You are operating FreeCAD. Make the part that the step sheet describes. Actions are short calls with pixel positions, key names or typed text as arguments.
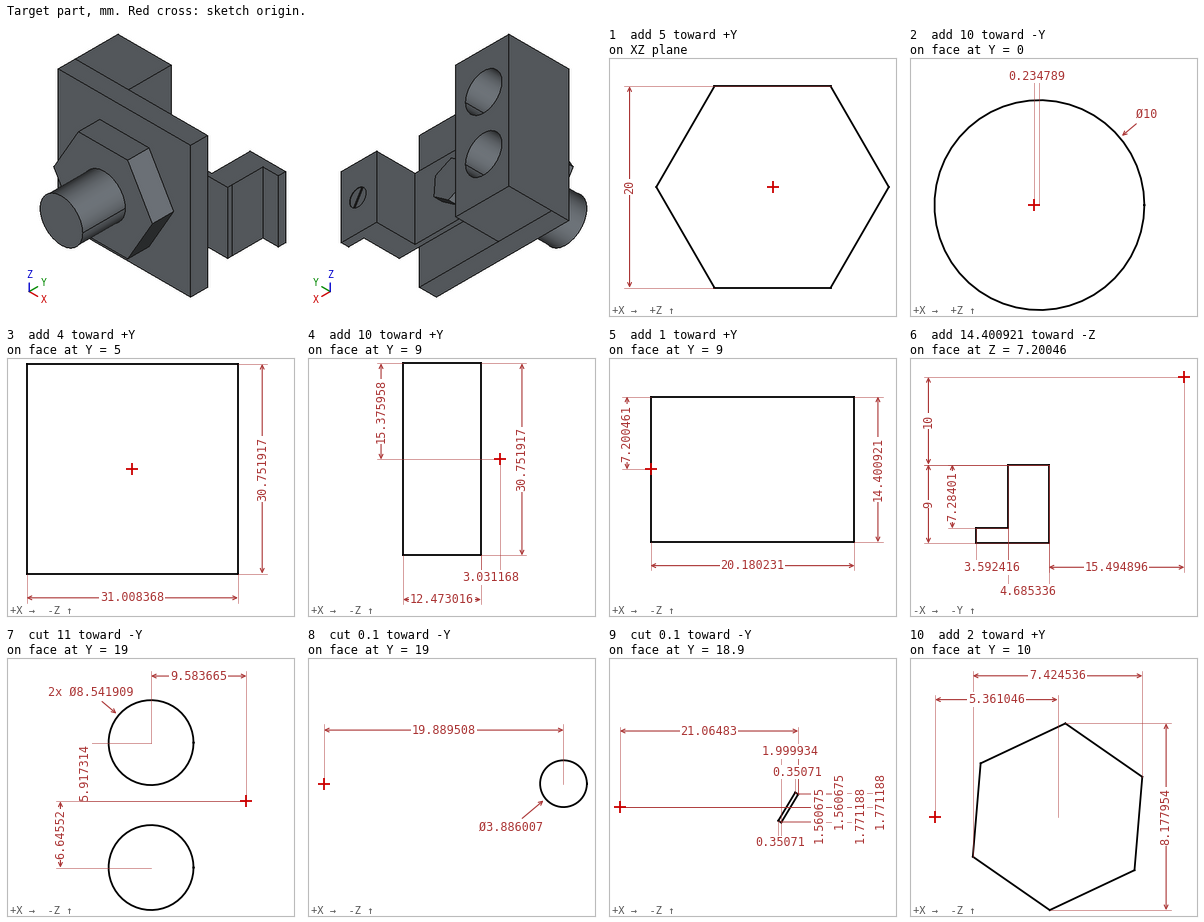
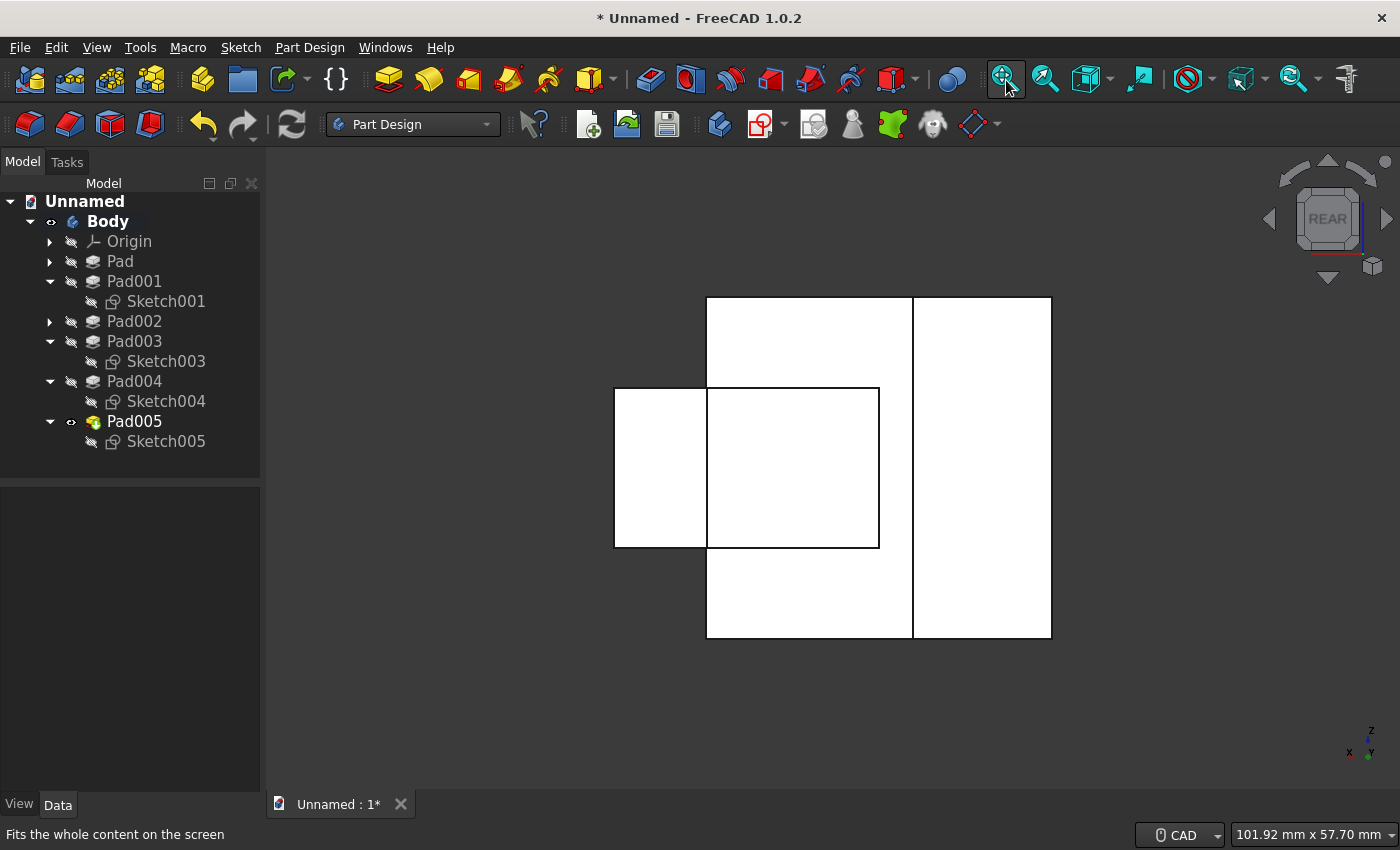
click(982, 516)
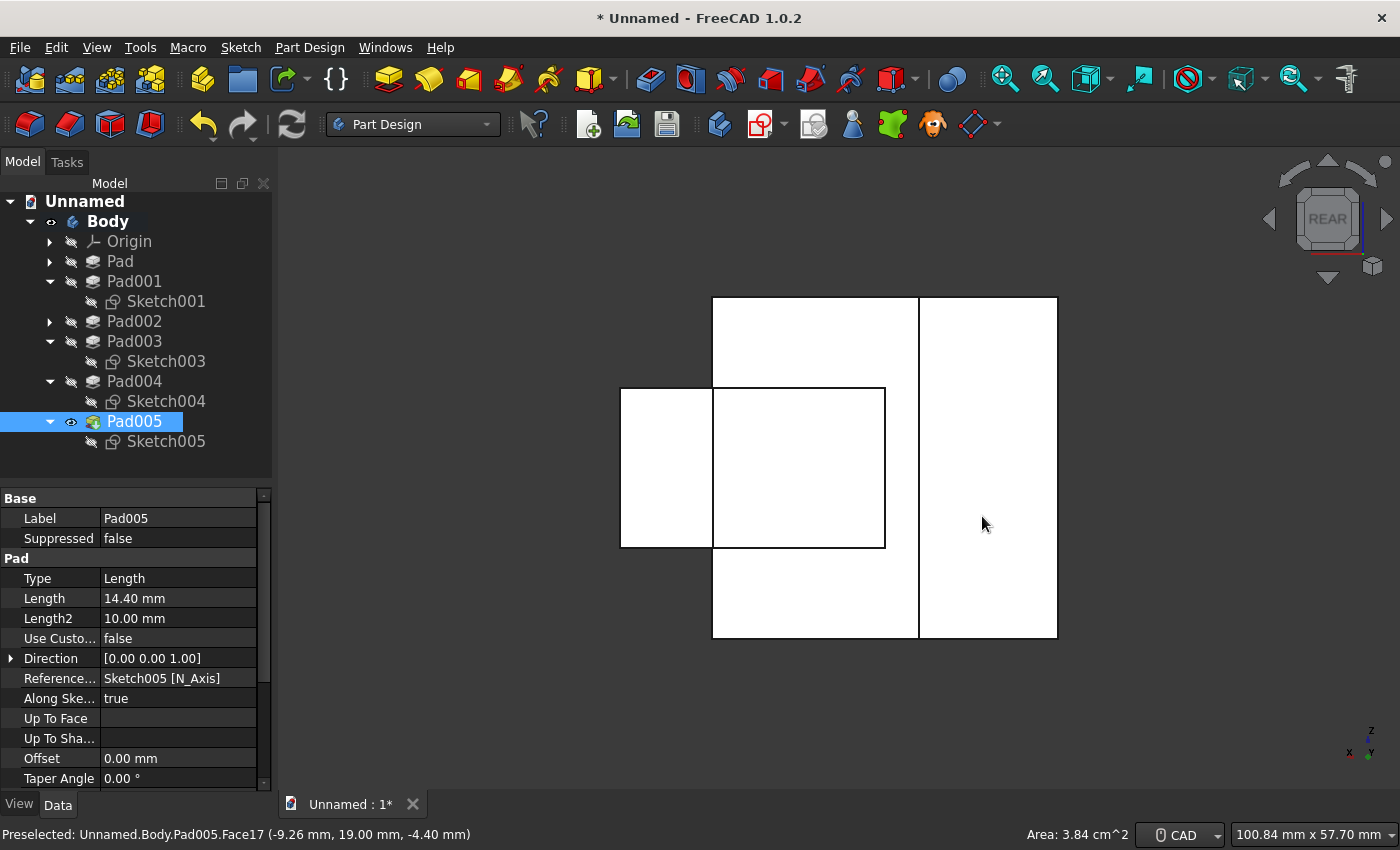
click(760, 124)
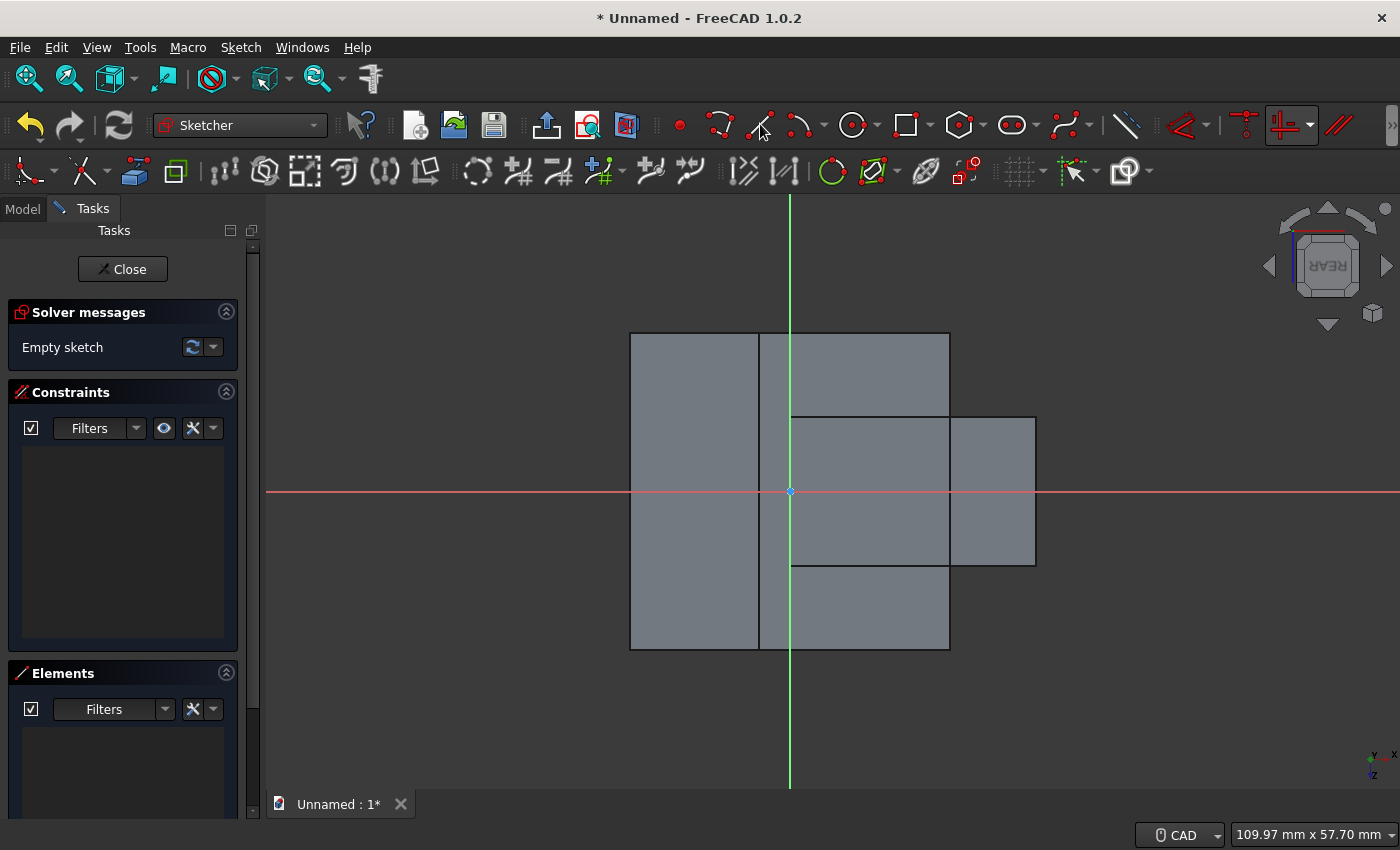
scroll(664, 500, up, 3)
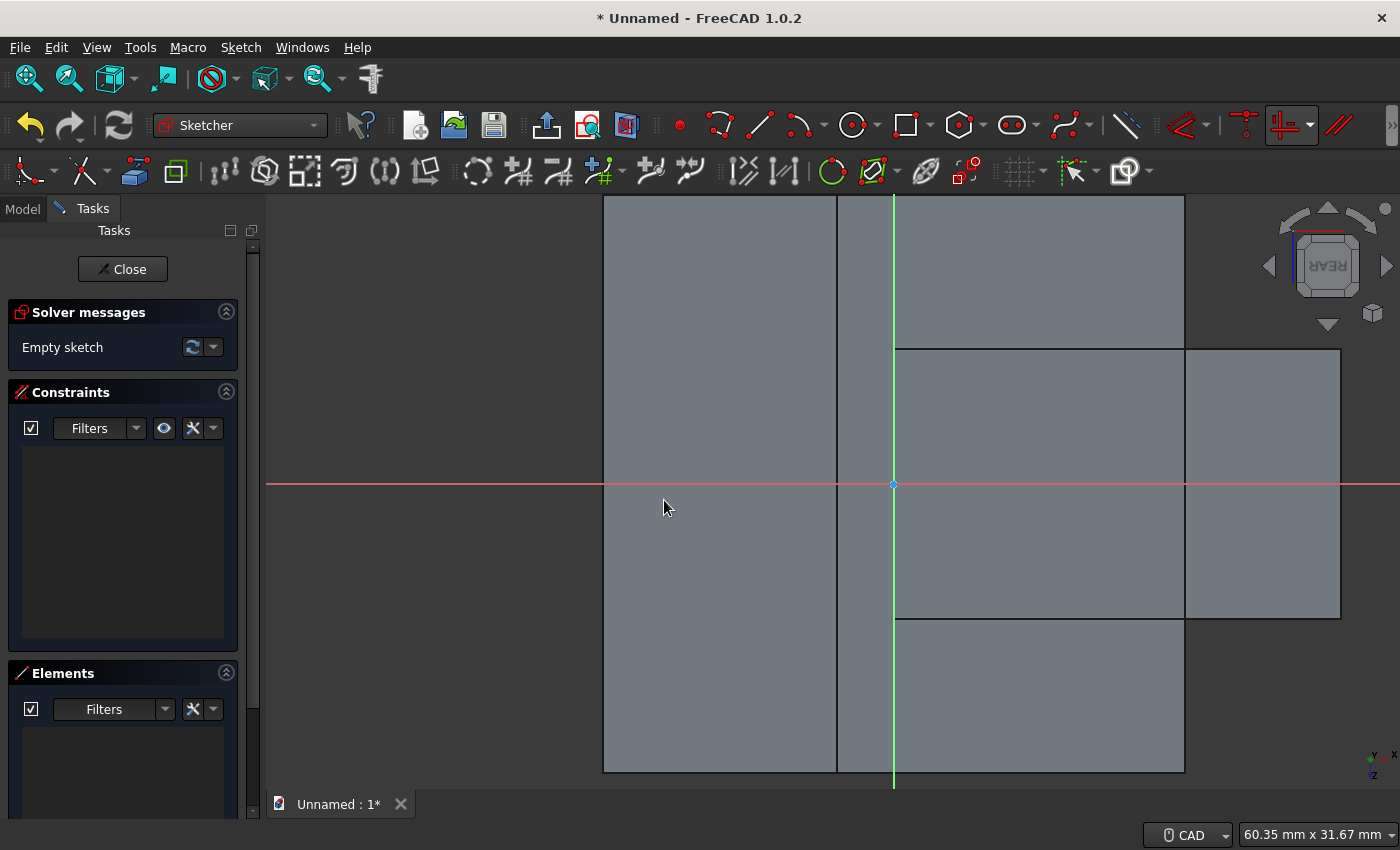
click(854, 126)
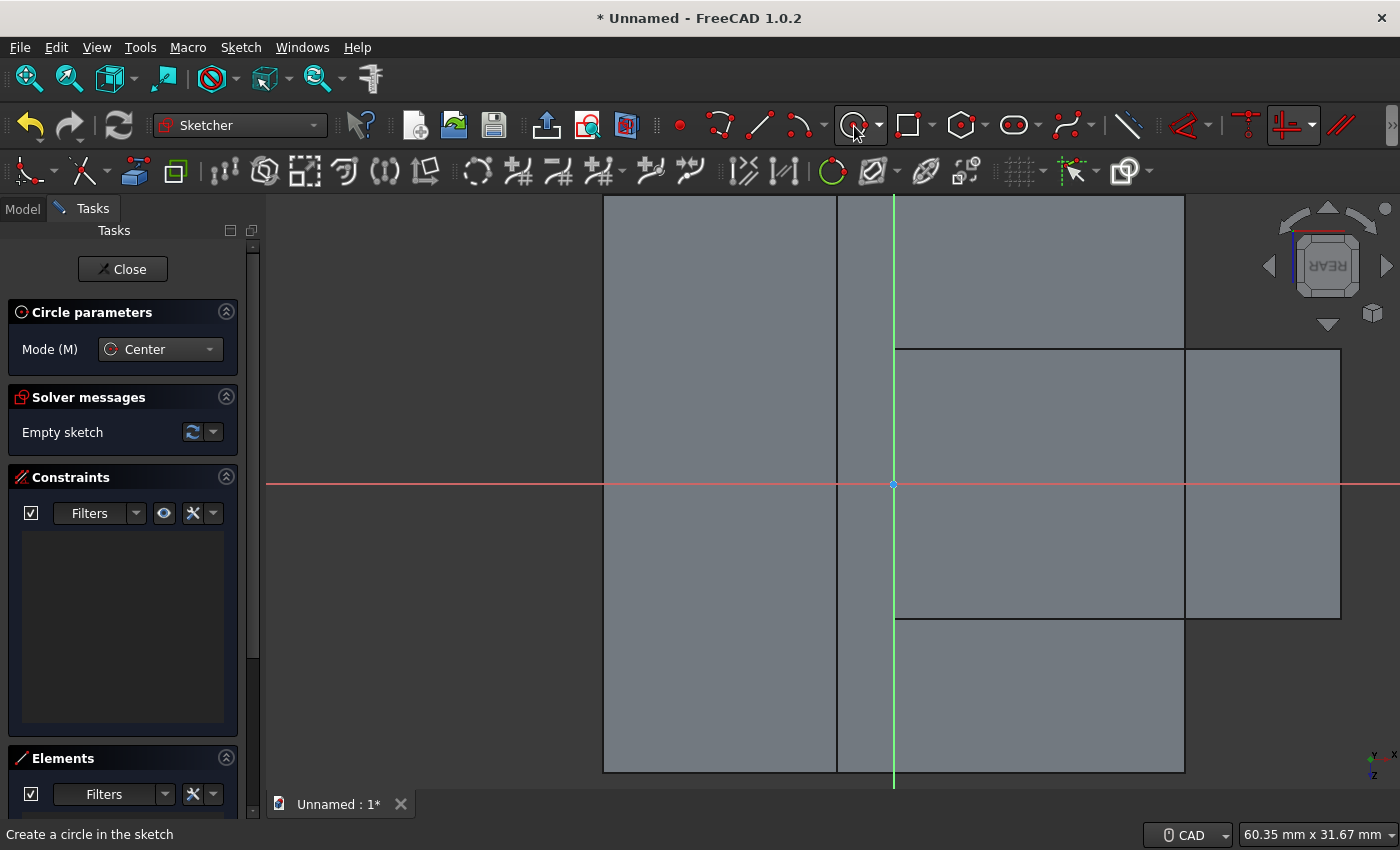
click(714, 373)
move(771, 316)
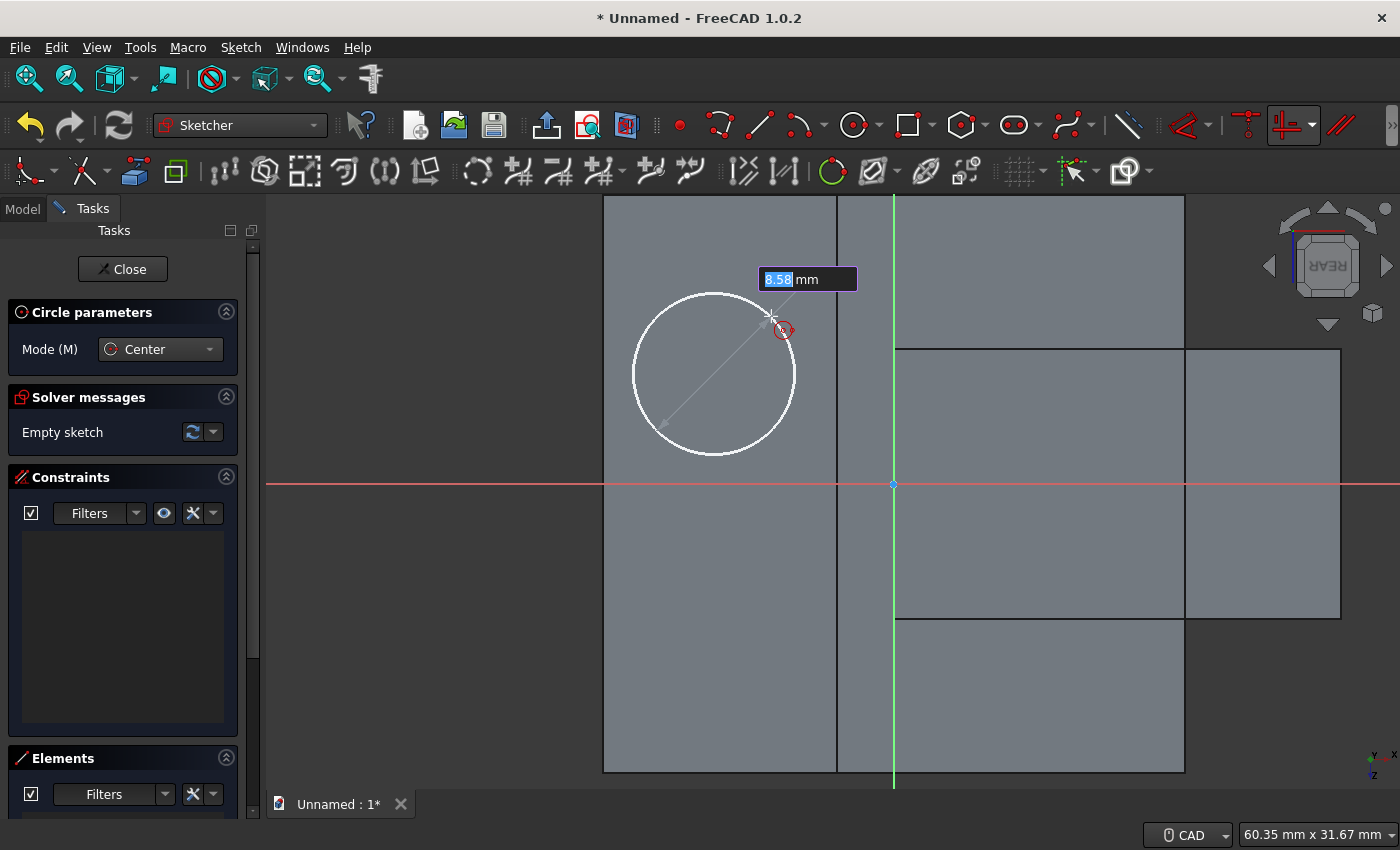
text(8.541909)
key(Return)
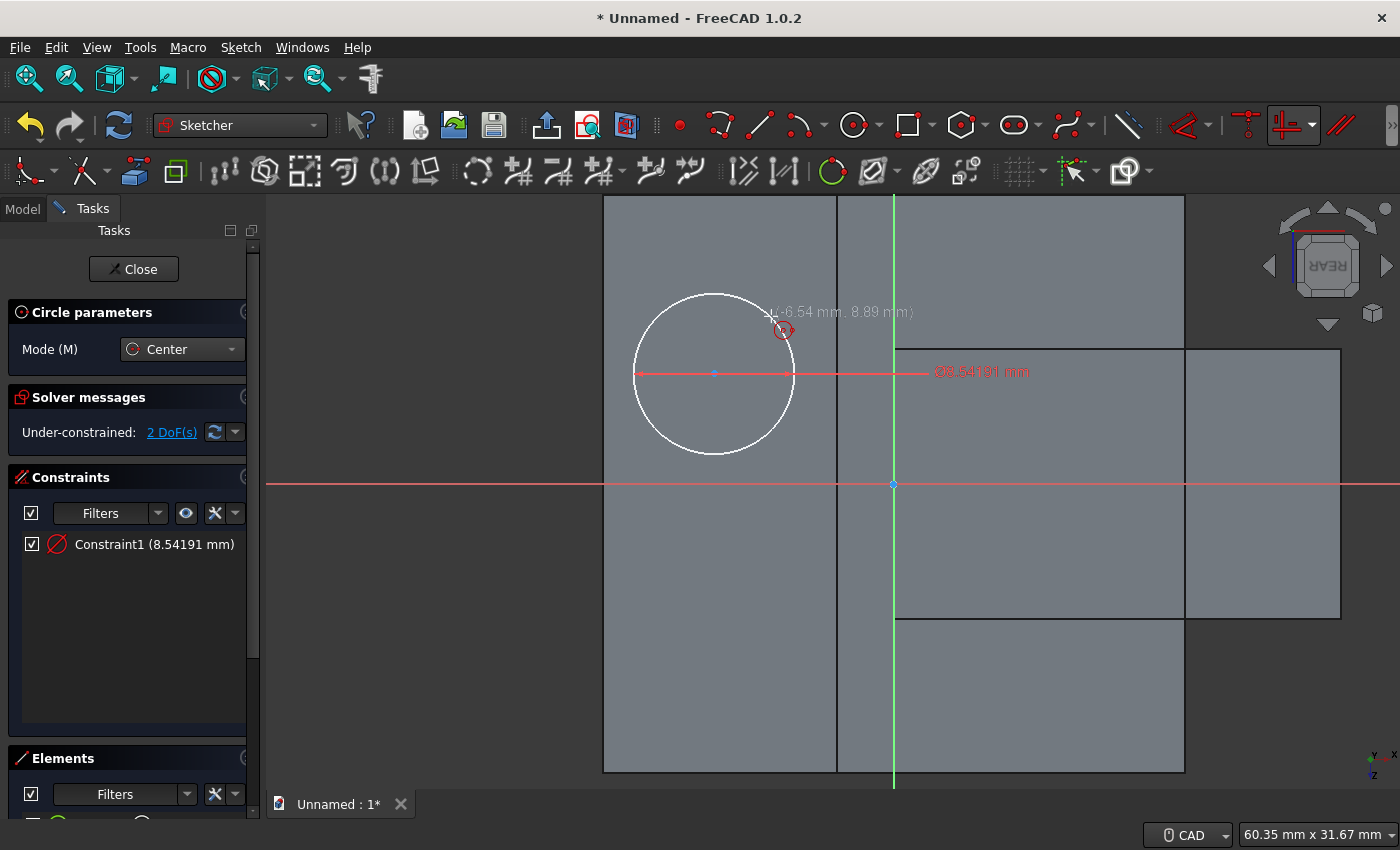
click(714, 609)
move(771, 552)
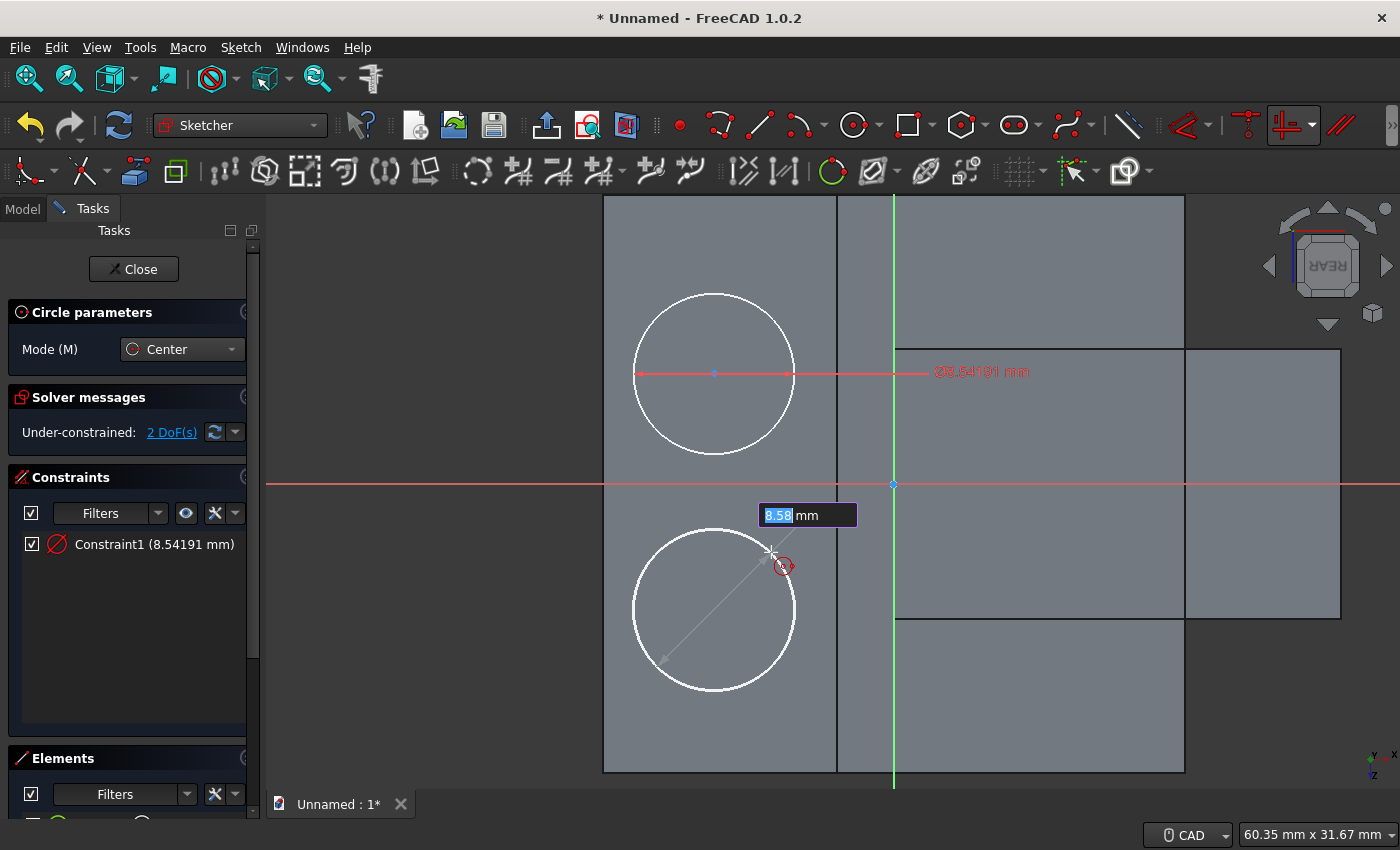
text(8.541909)
key(Return)
key(Escape)